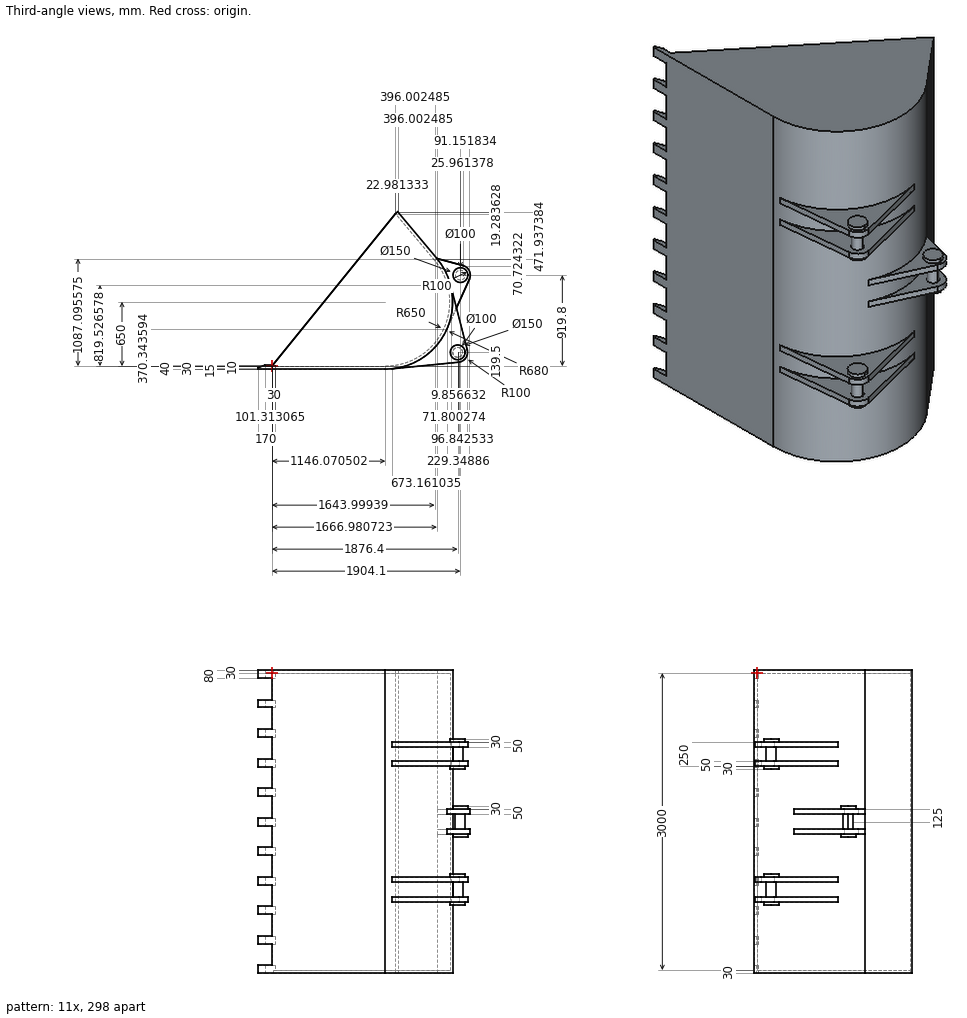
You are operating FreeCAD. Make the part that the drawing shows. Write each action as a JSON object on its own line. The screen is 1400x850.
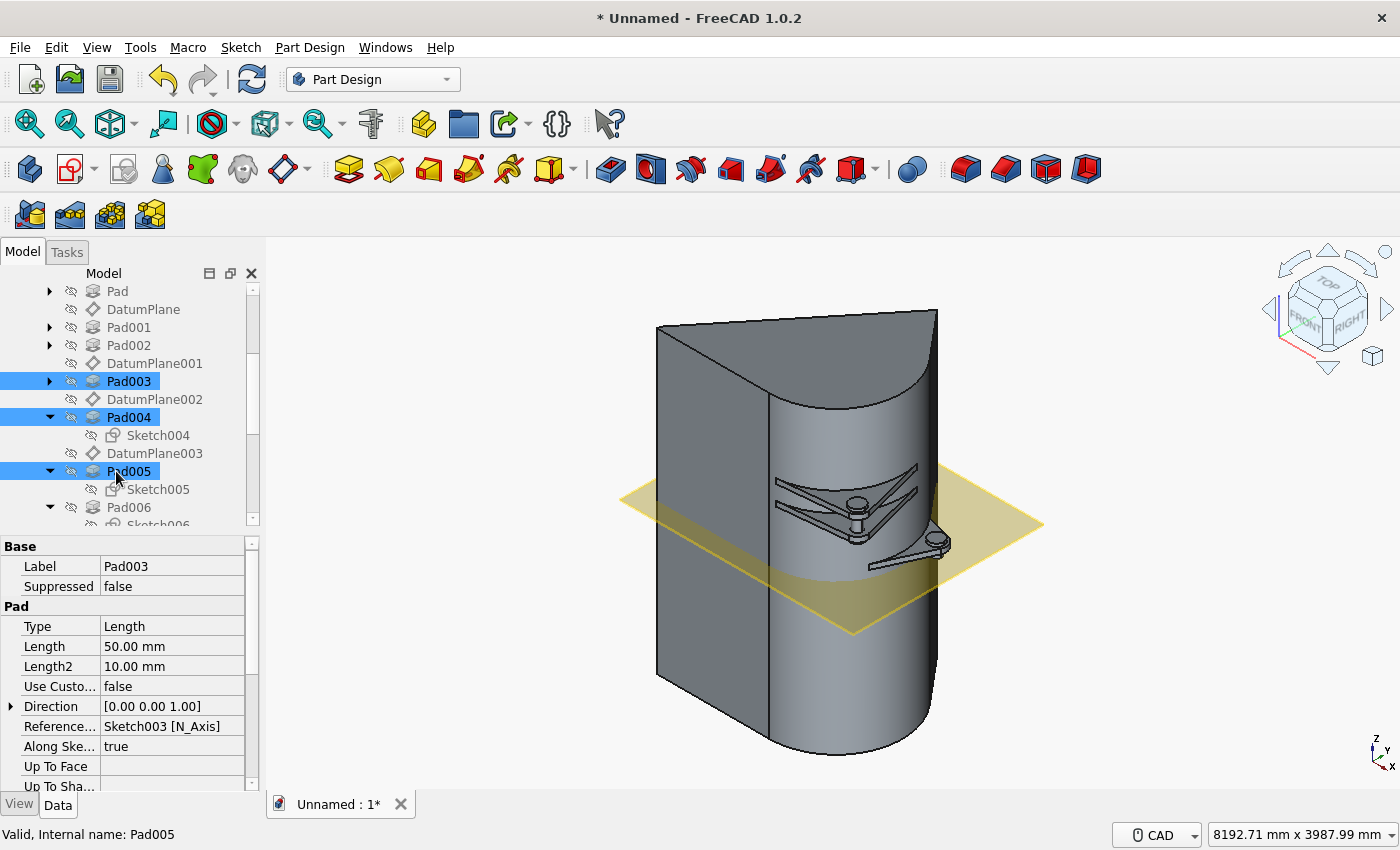
{"action": "left_click", "coordinate": [116, 507], "text": "ctrl"}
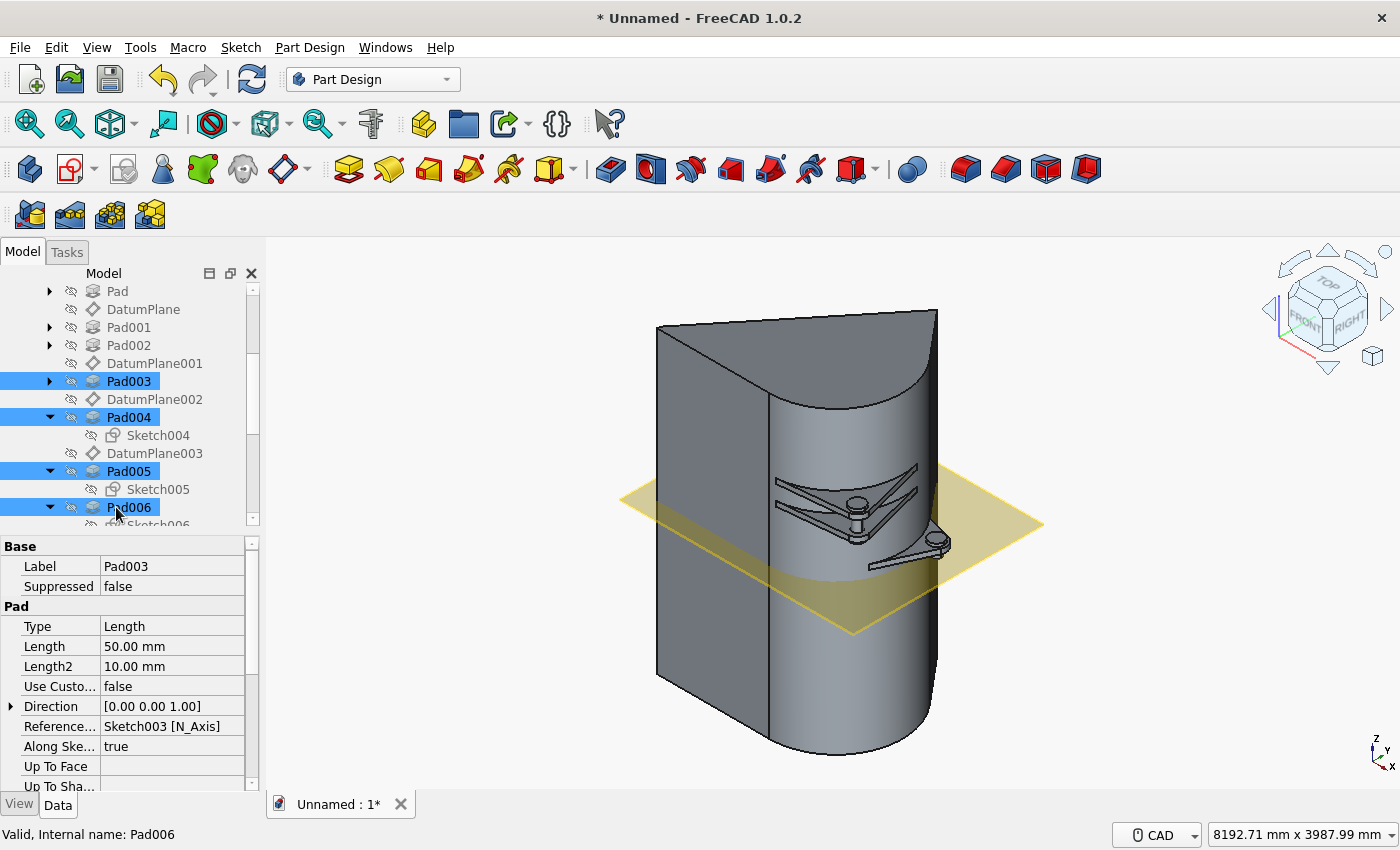
{"action": "scroll", "coordinate": [140, 413], "scroll_direction": "down", "scroll_amount": 3}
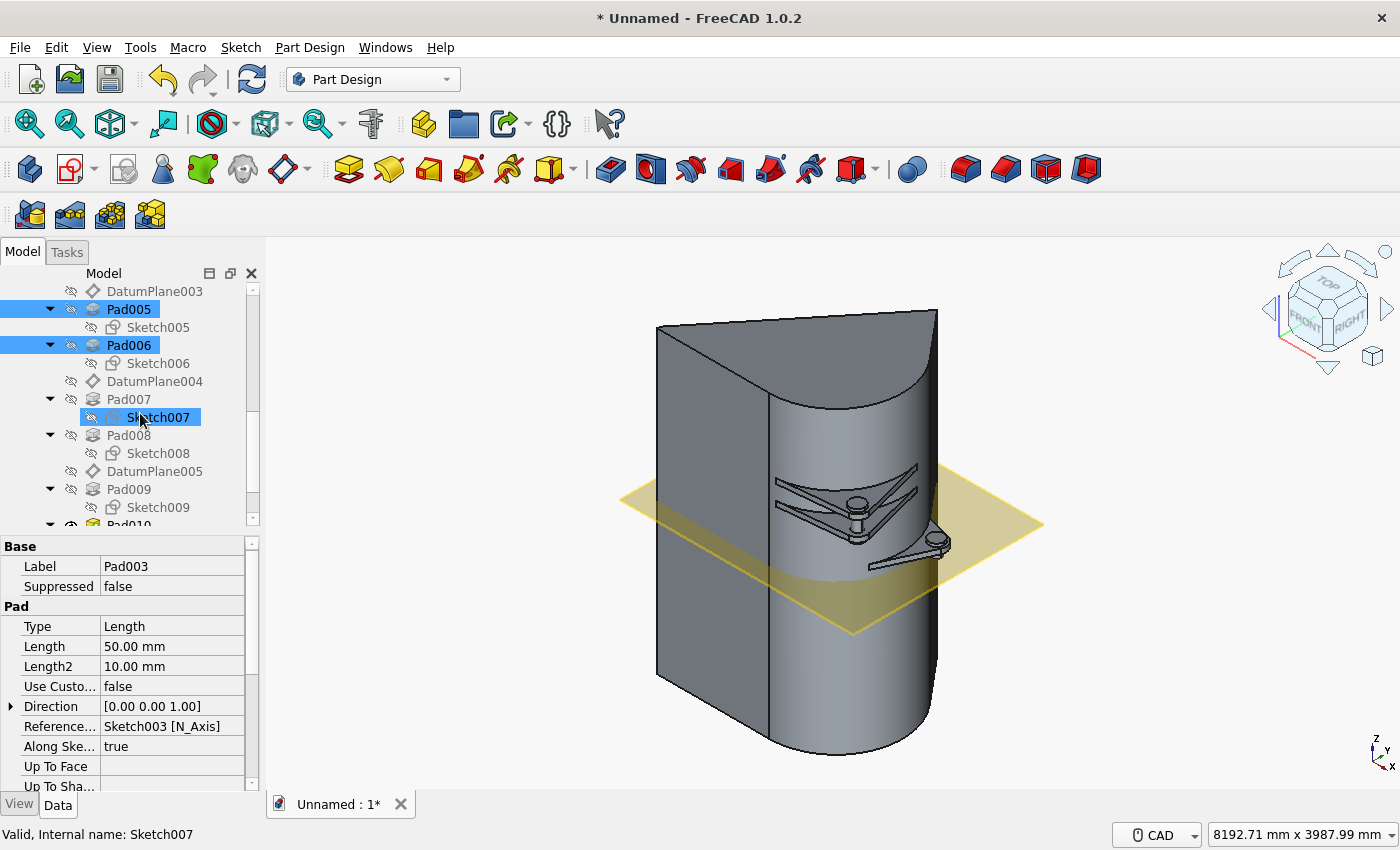
{"action": "left_click", "coordinate": [116, 399], "text": "ctrl"}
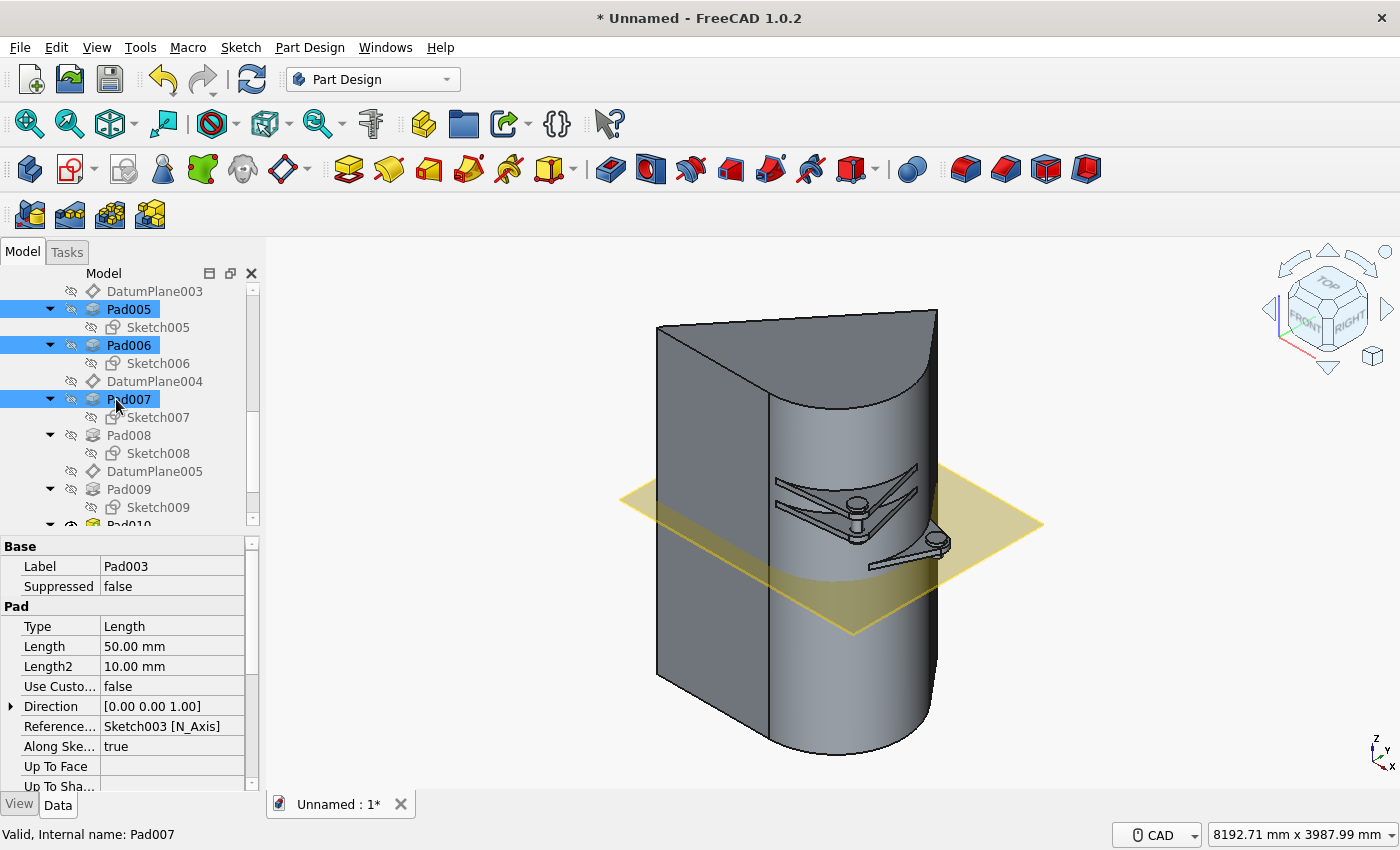
{"action": "left_click", "coordinate": [116, 435], "text": "ctrl"}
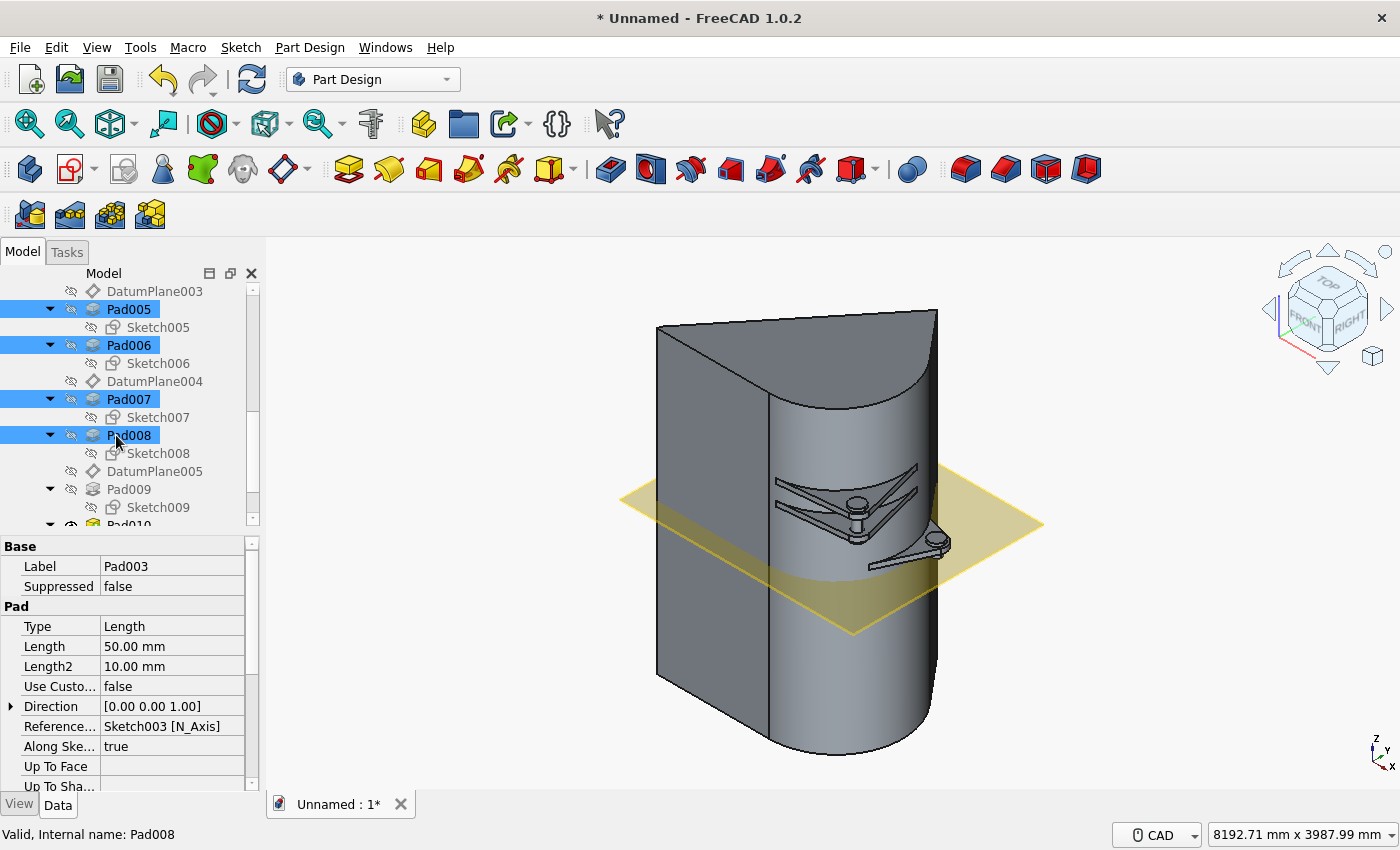
{"action": "left_click", "coordinate": [116, 489], "text": "ctrl"}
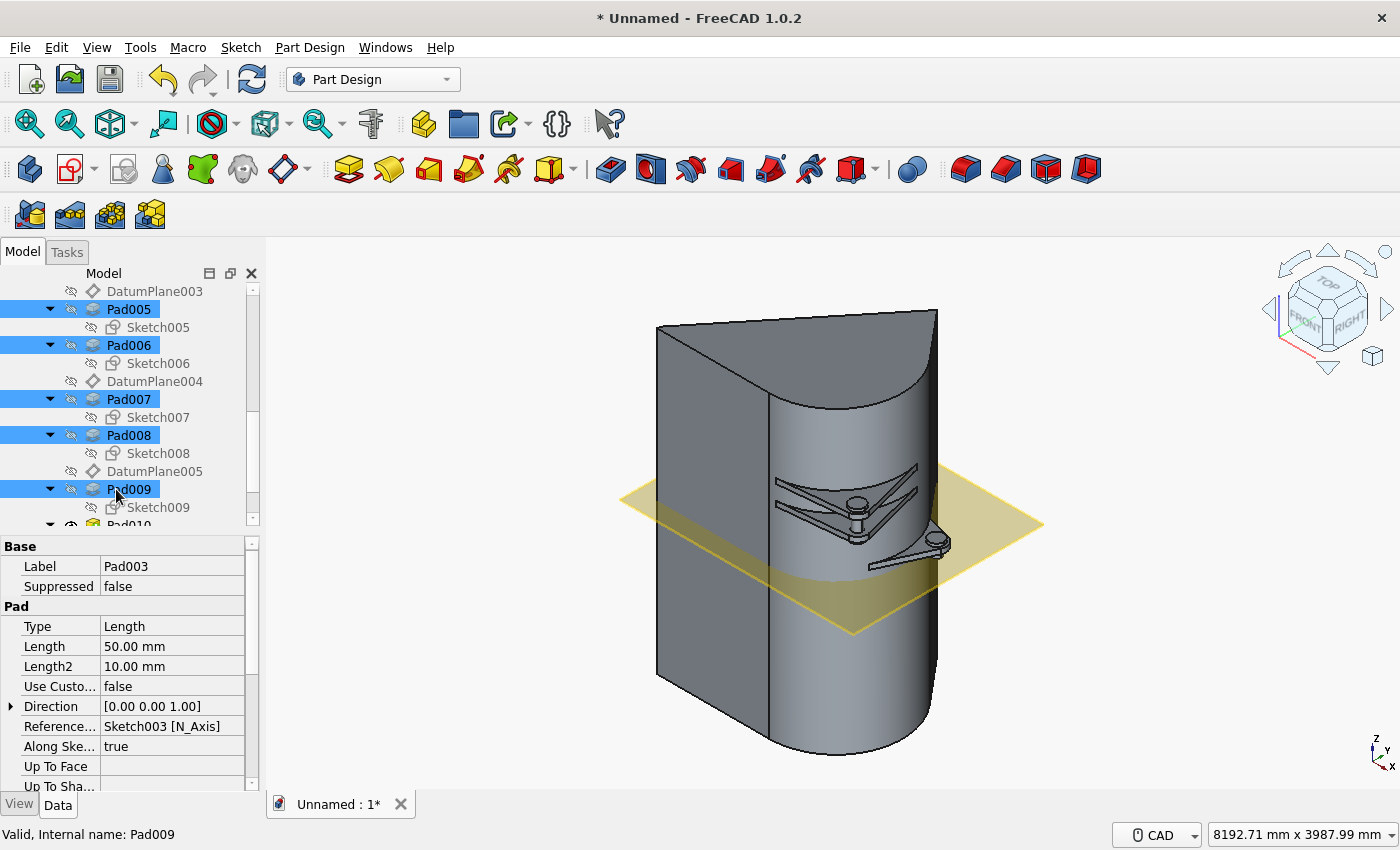
{"action": "left_click", "coordinate": [116, 525], "text": "ctrl"}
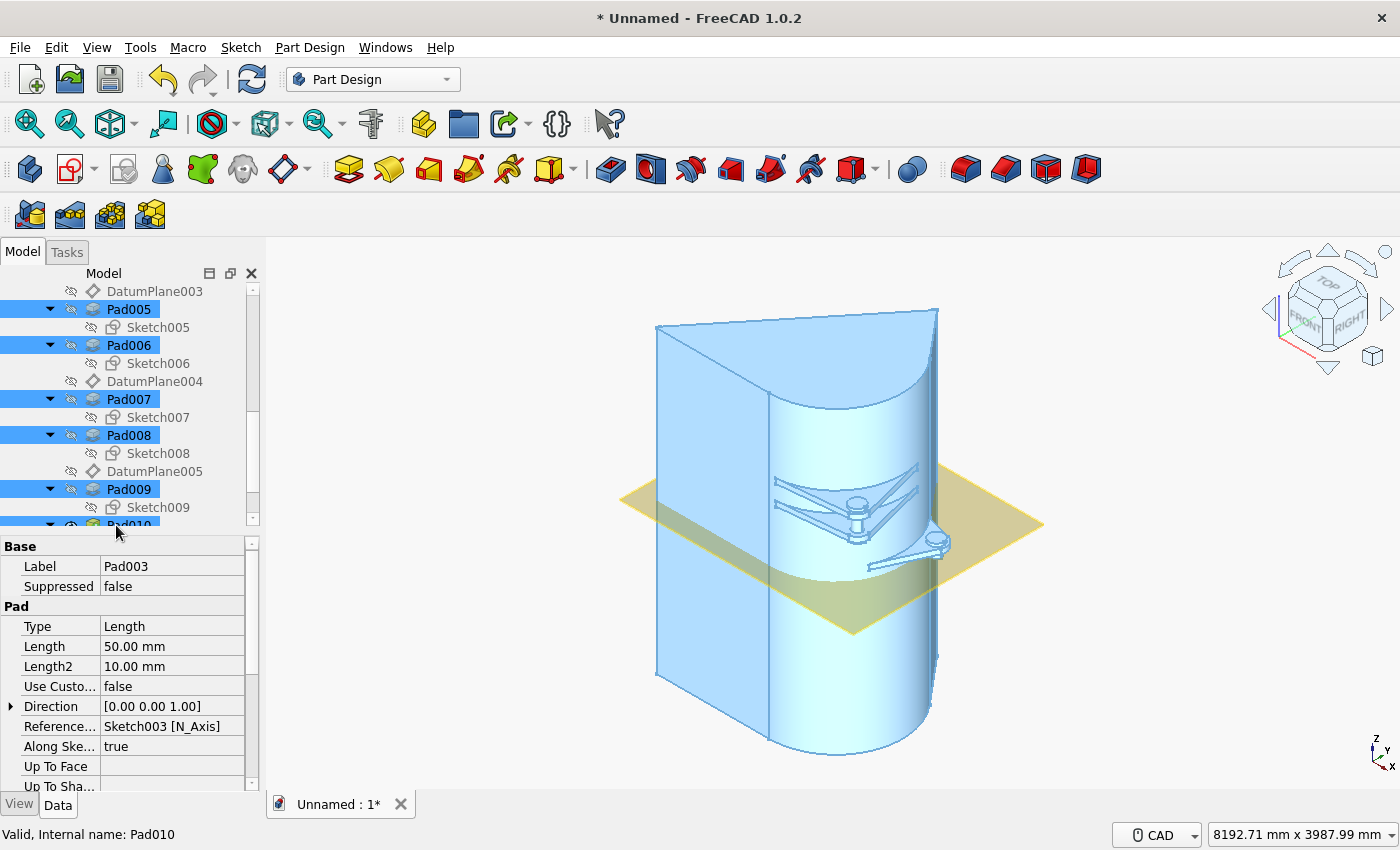
{"action": "left_click", "coordinate": [30, 214]}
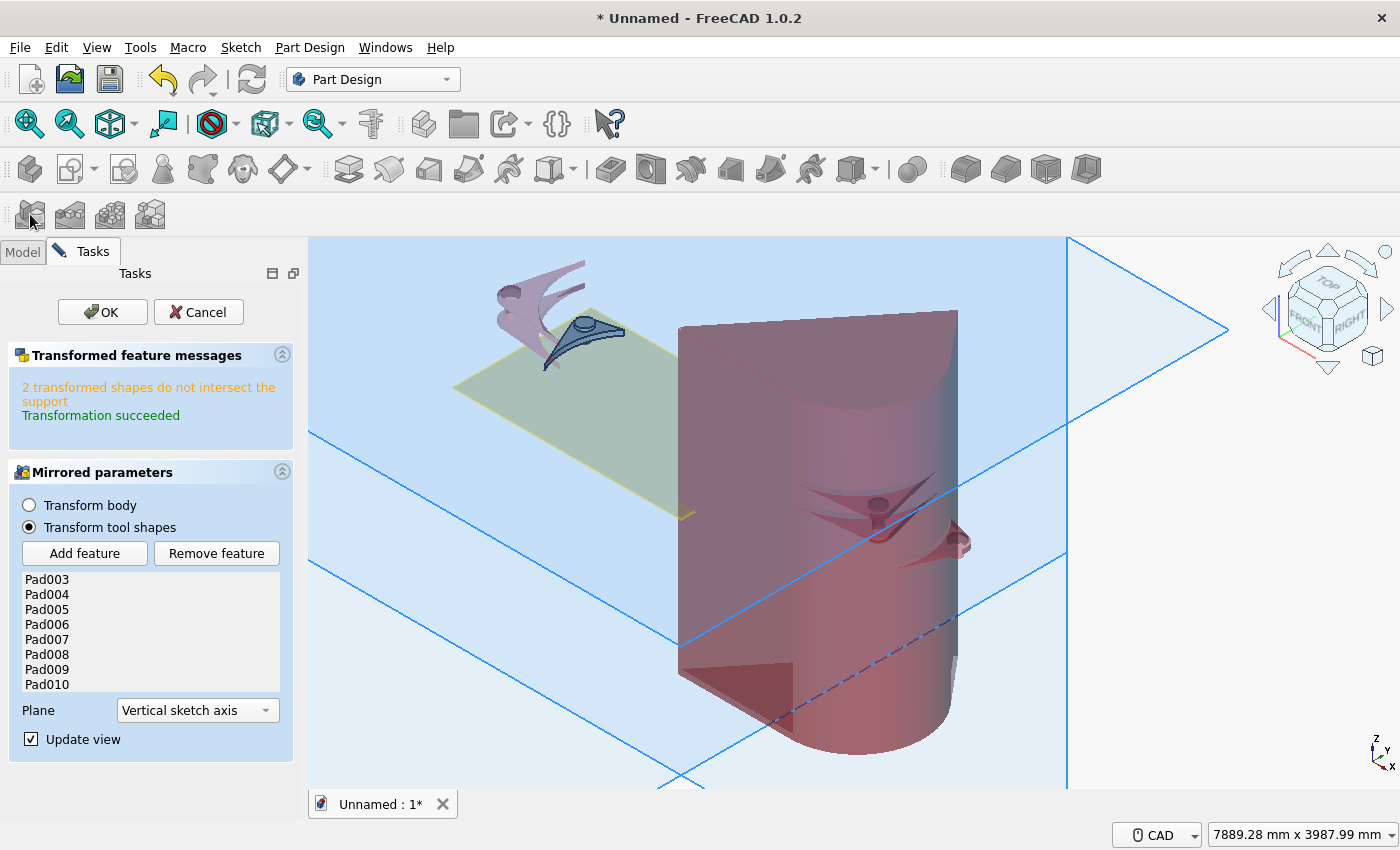
{"action": "left_click", "coordinate": [198, 710]}